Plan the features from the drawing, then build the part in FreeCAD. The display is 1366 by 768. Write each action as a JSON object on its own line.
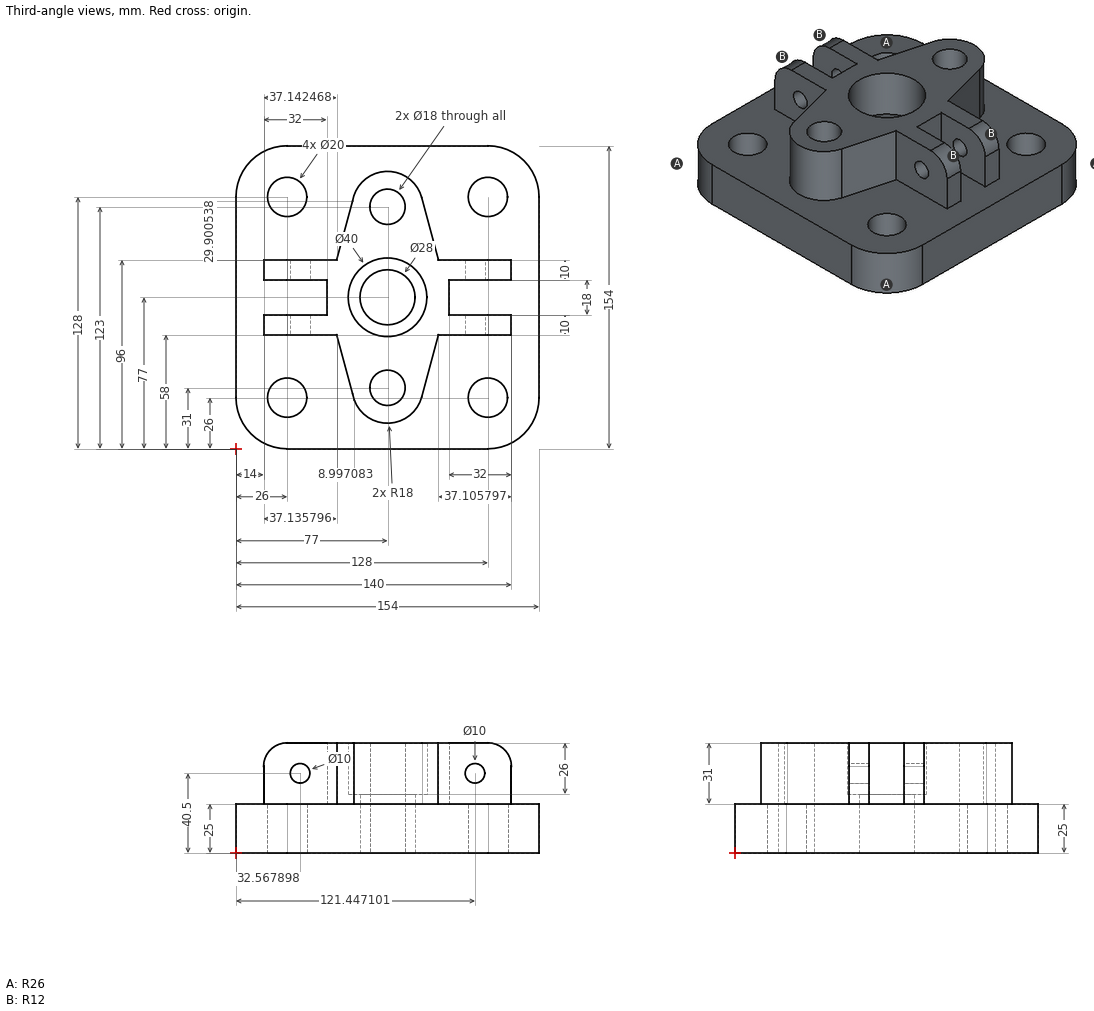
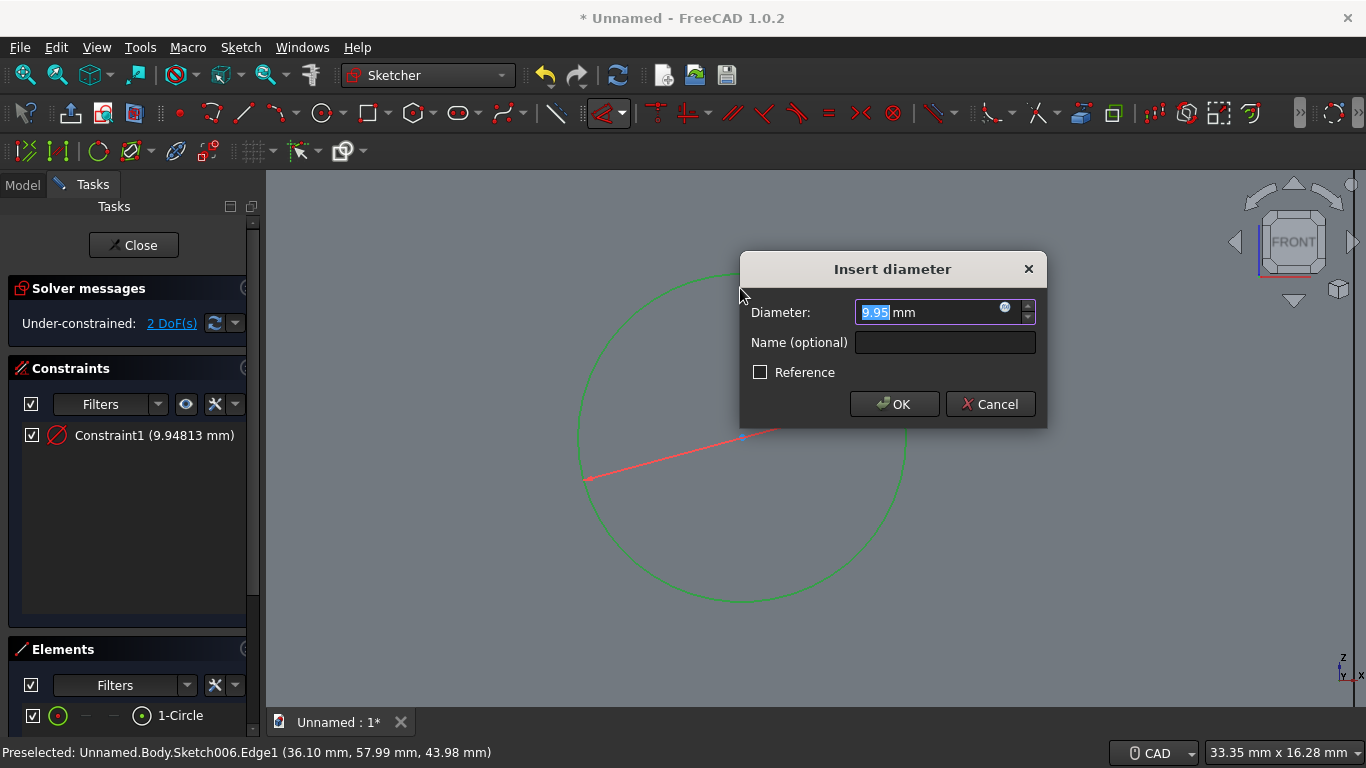
{"action": "type", "text": "10"}
{"action": "key", "text": "Return"}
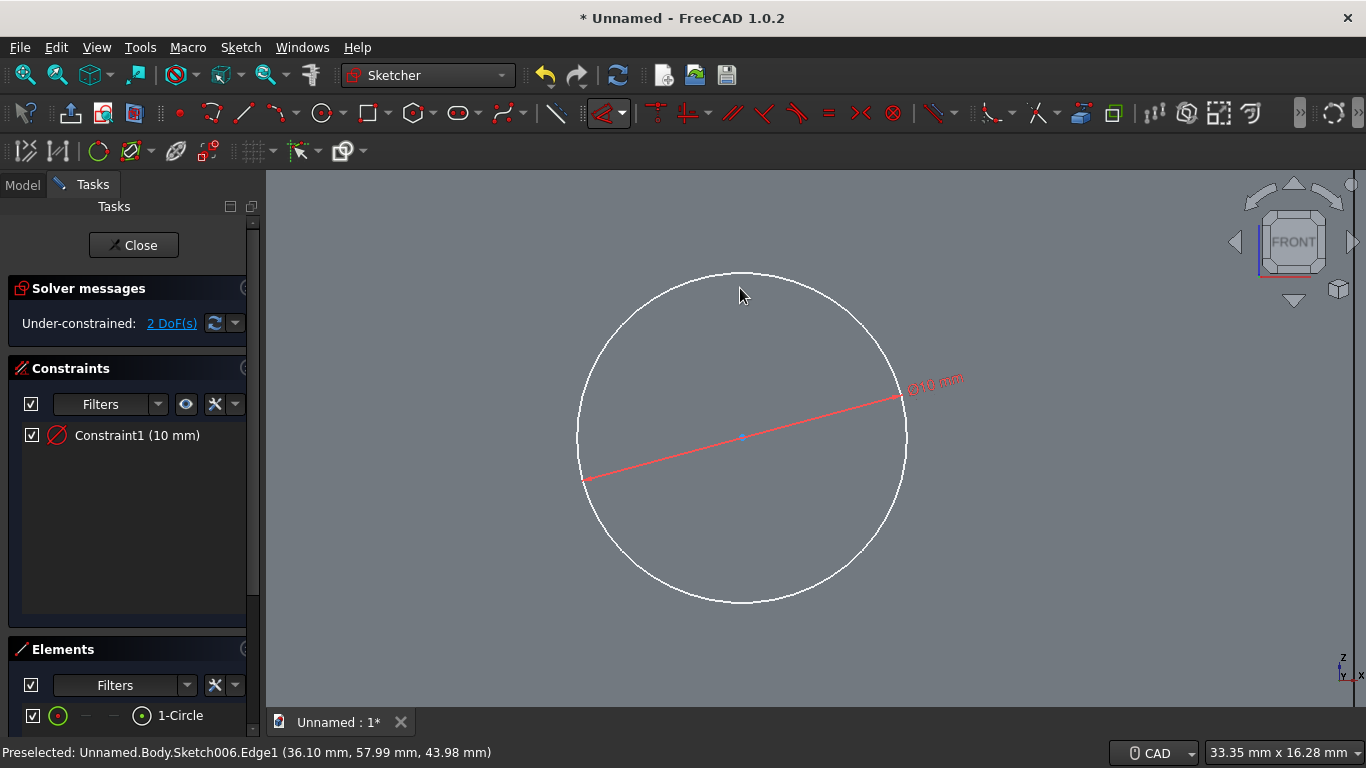
{"action": "left_click", "coordinate": [742, 438]}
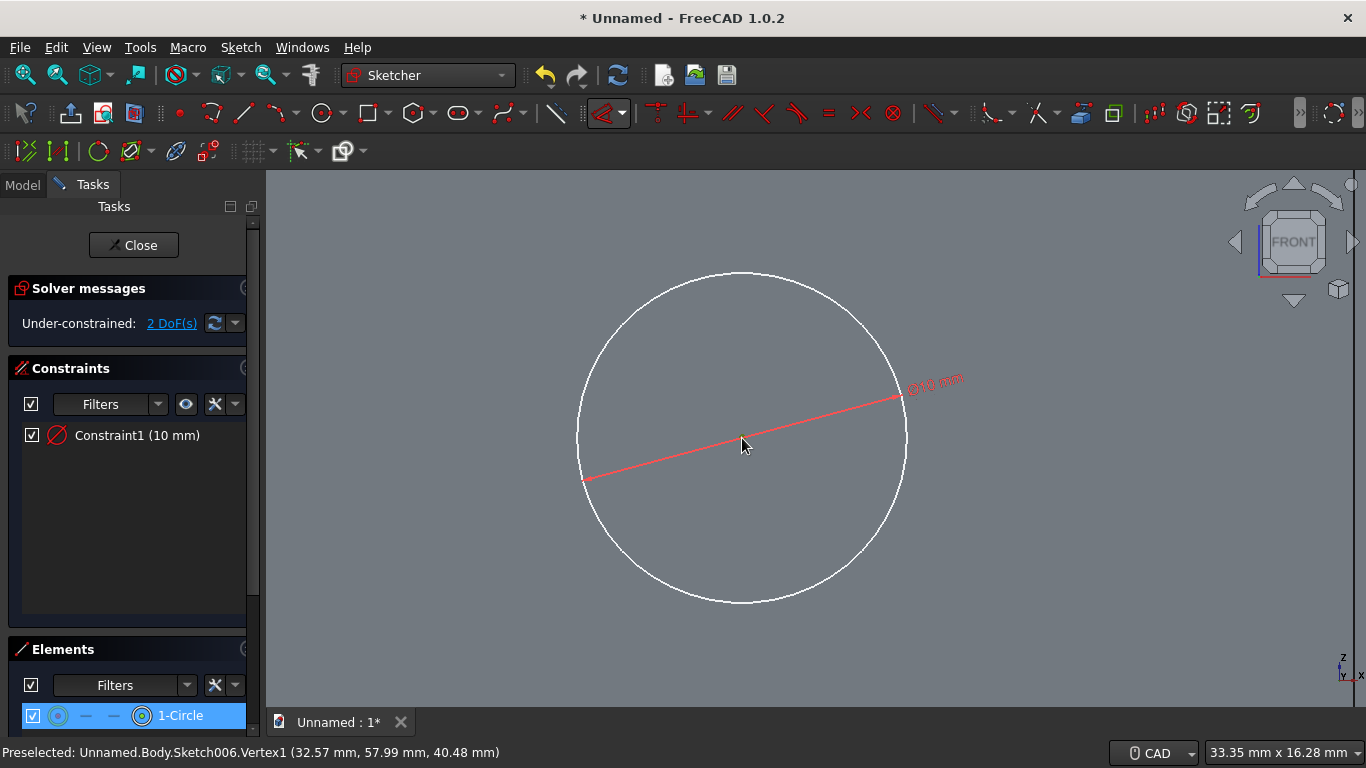
{"action": "key", "text": "i"}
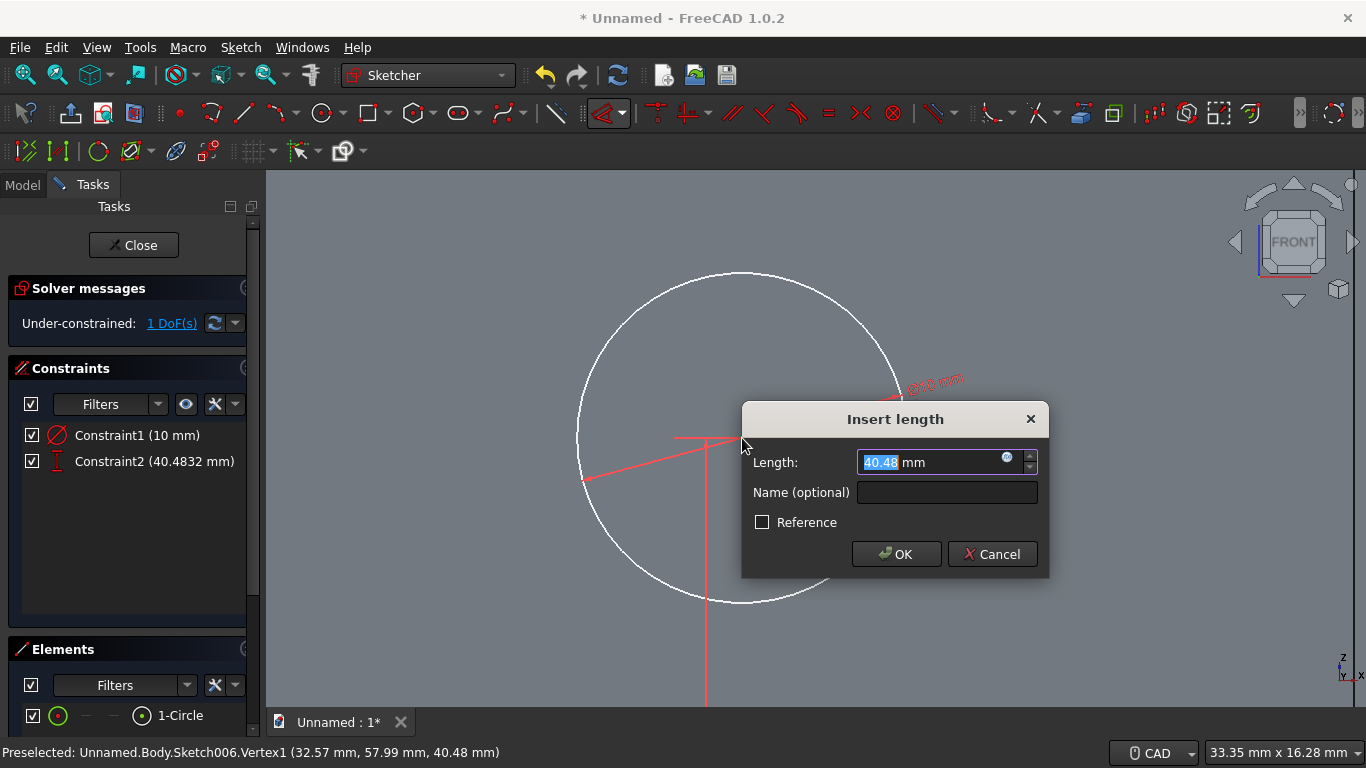
{"action": "type", "text": "40.5"}
{"action": "key", "text": "Return"}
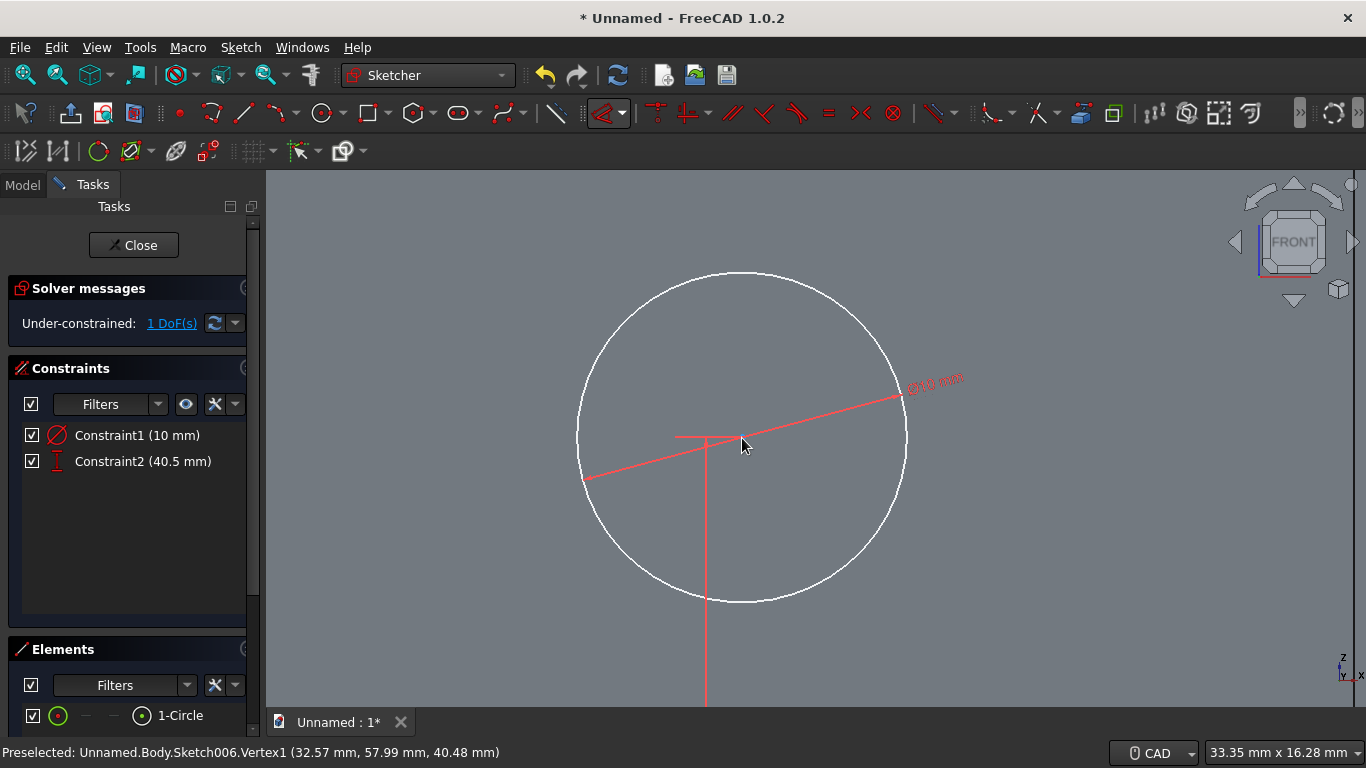
{"action": "left_click", "coordinate": [742, 437]}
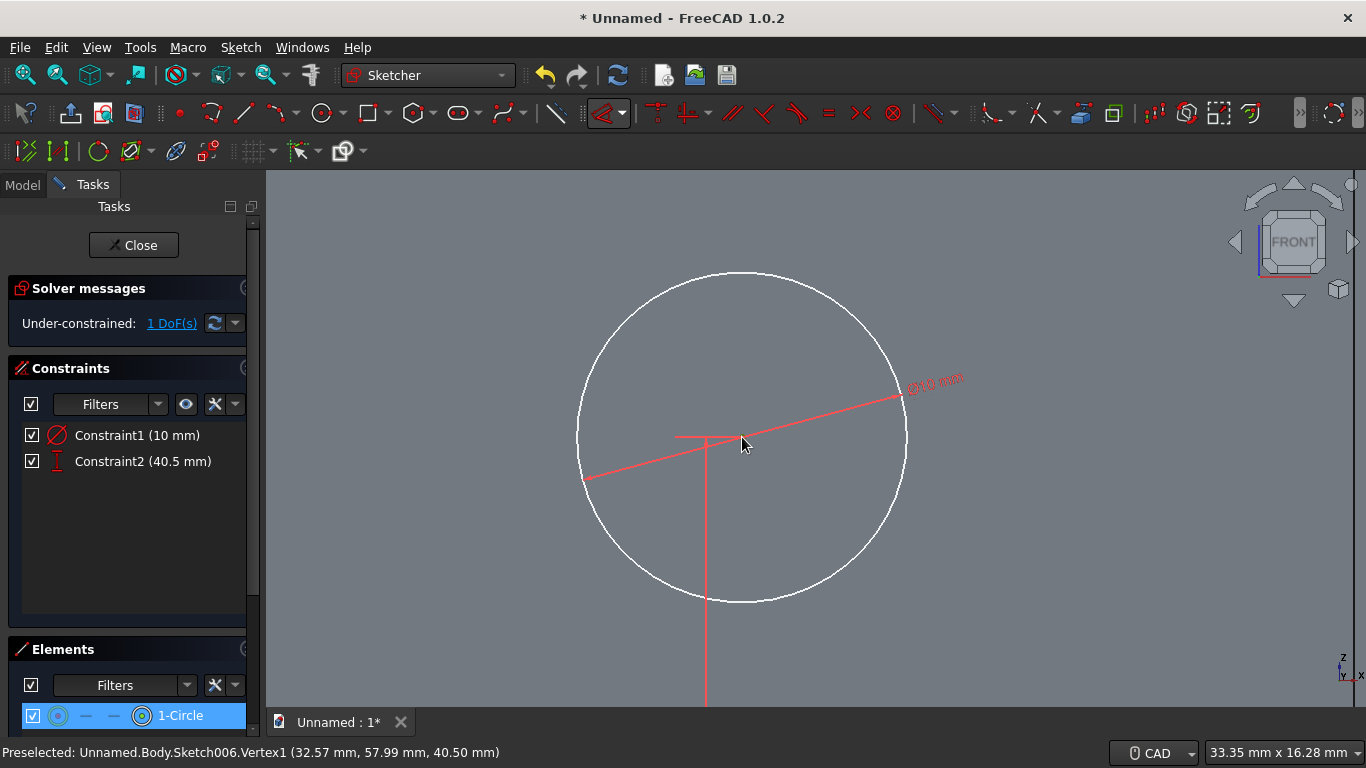
{"action": "key", "text": "l"}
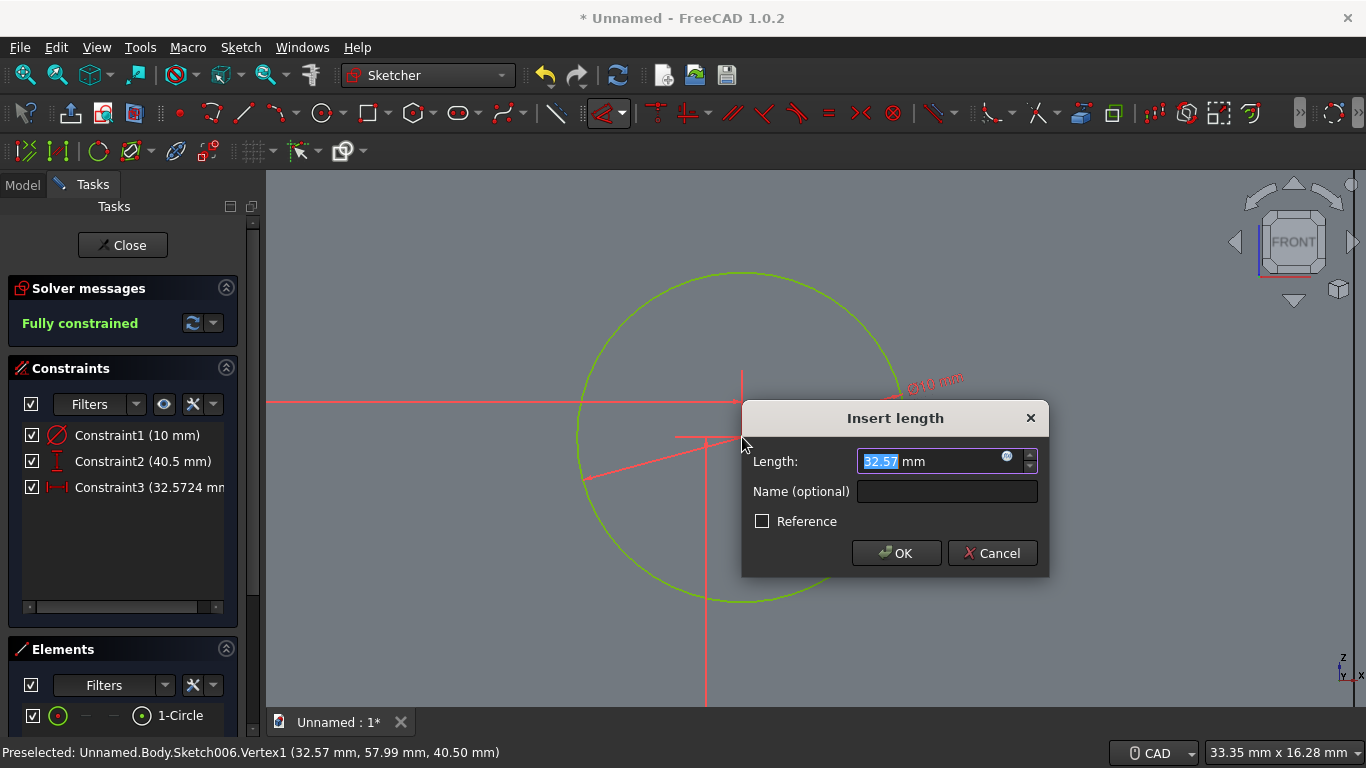
{"action": "type", "text": "32.567898"}
{"action": "key", "text": "Return"}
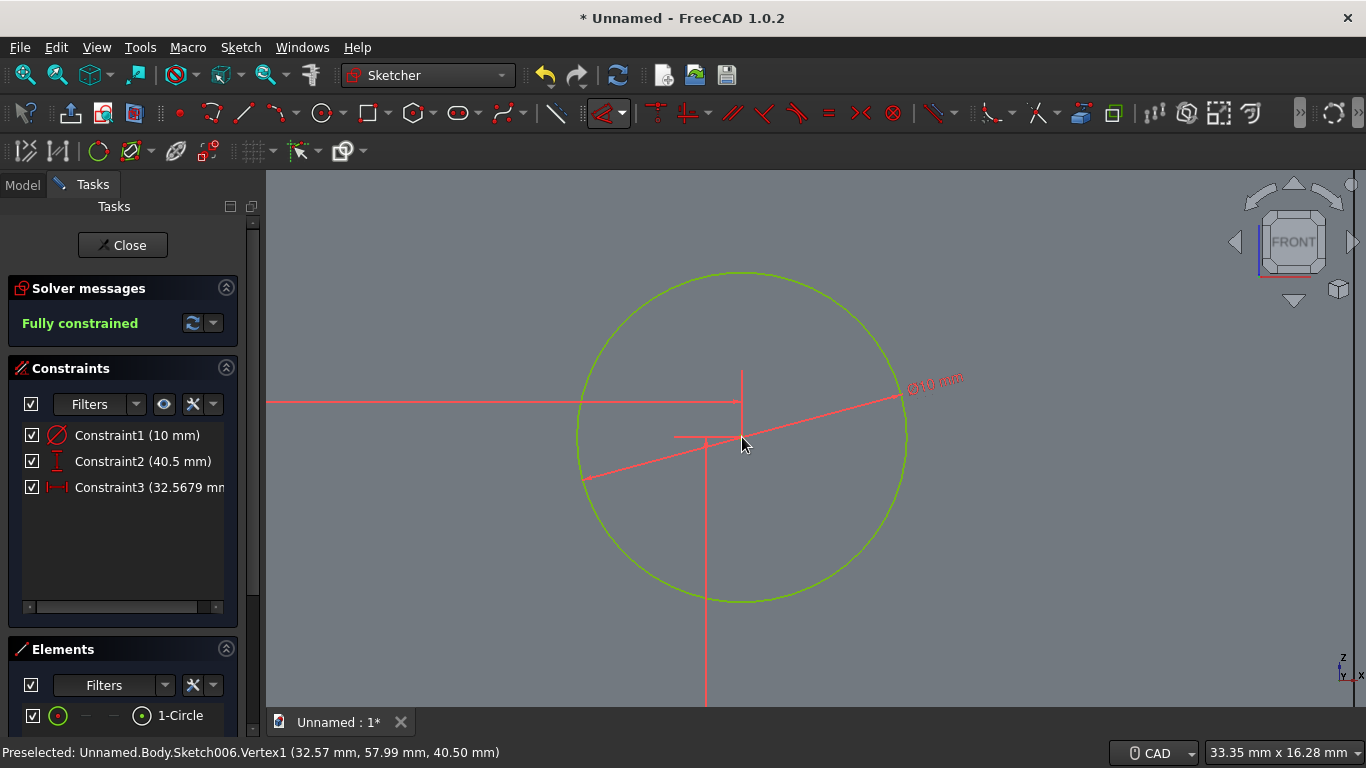
{"action": "left_click", "coordinate": [123, 245]}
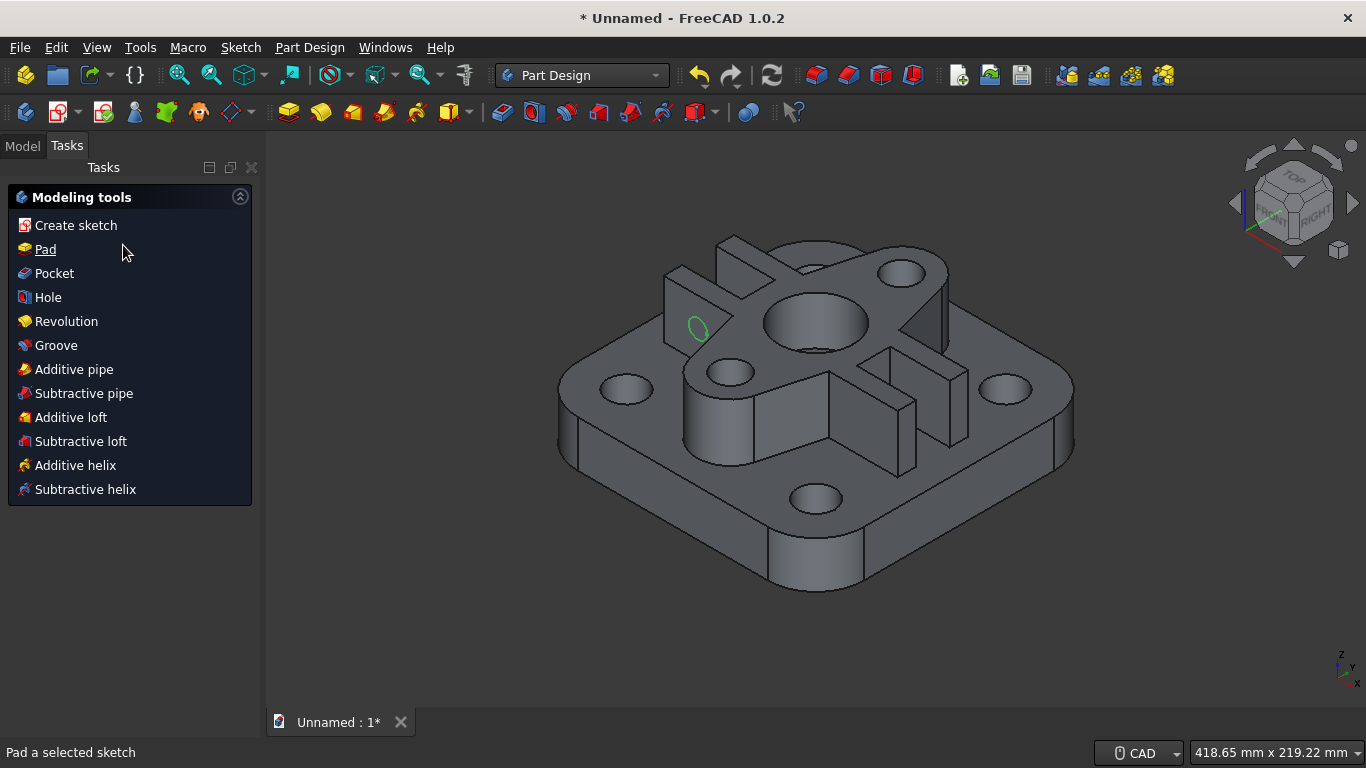
{"action": "left_click", "coordinate": [504, 112]}